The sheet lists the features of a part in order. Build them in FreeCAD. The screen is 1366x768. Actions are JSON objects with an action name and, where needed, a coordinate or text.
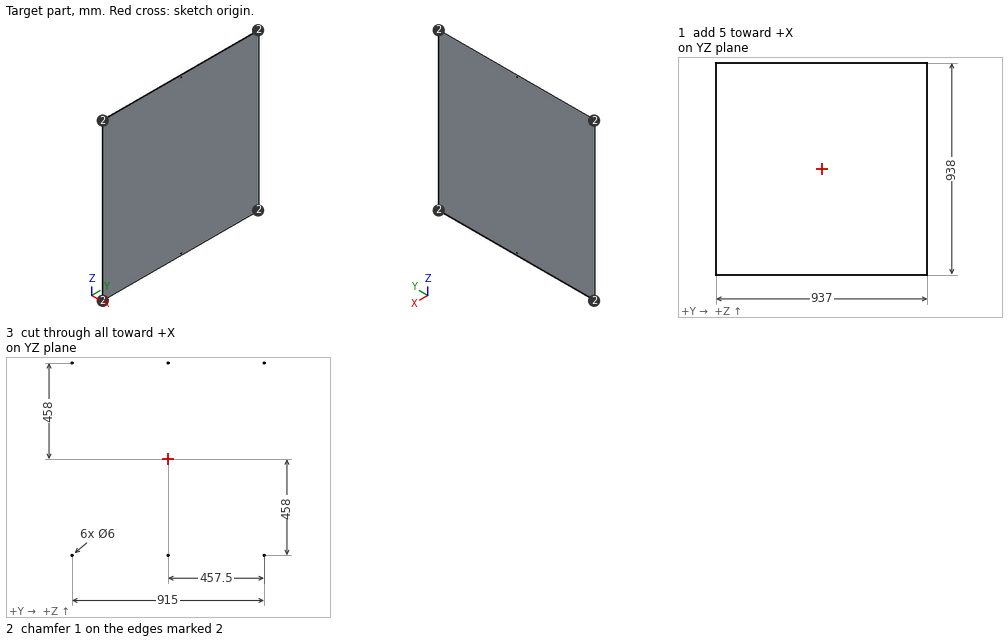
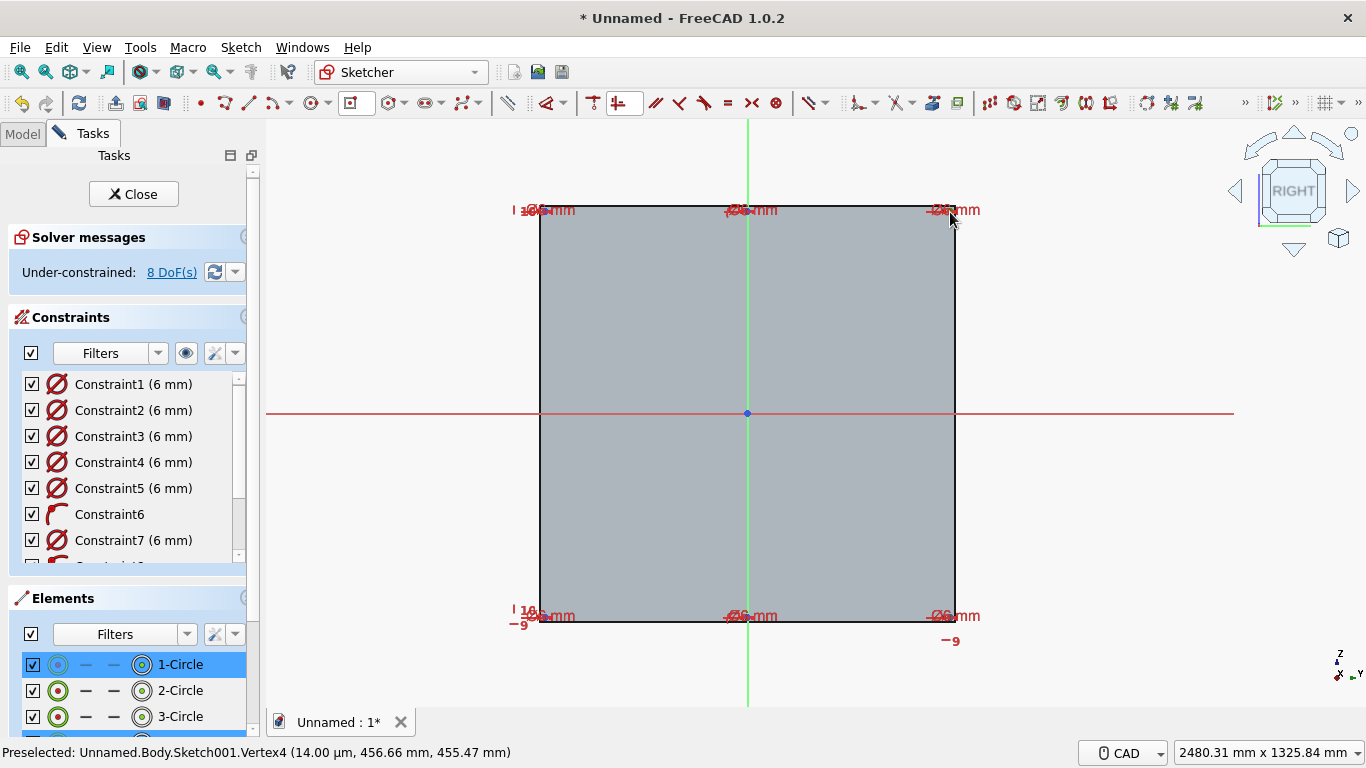
{"action": "key", "text": "v"}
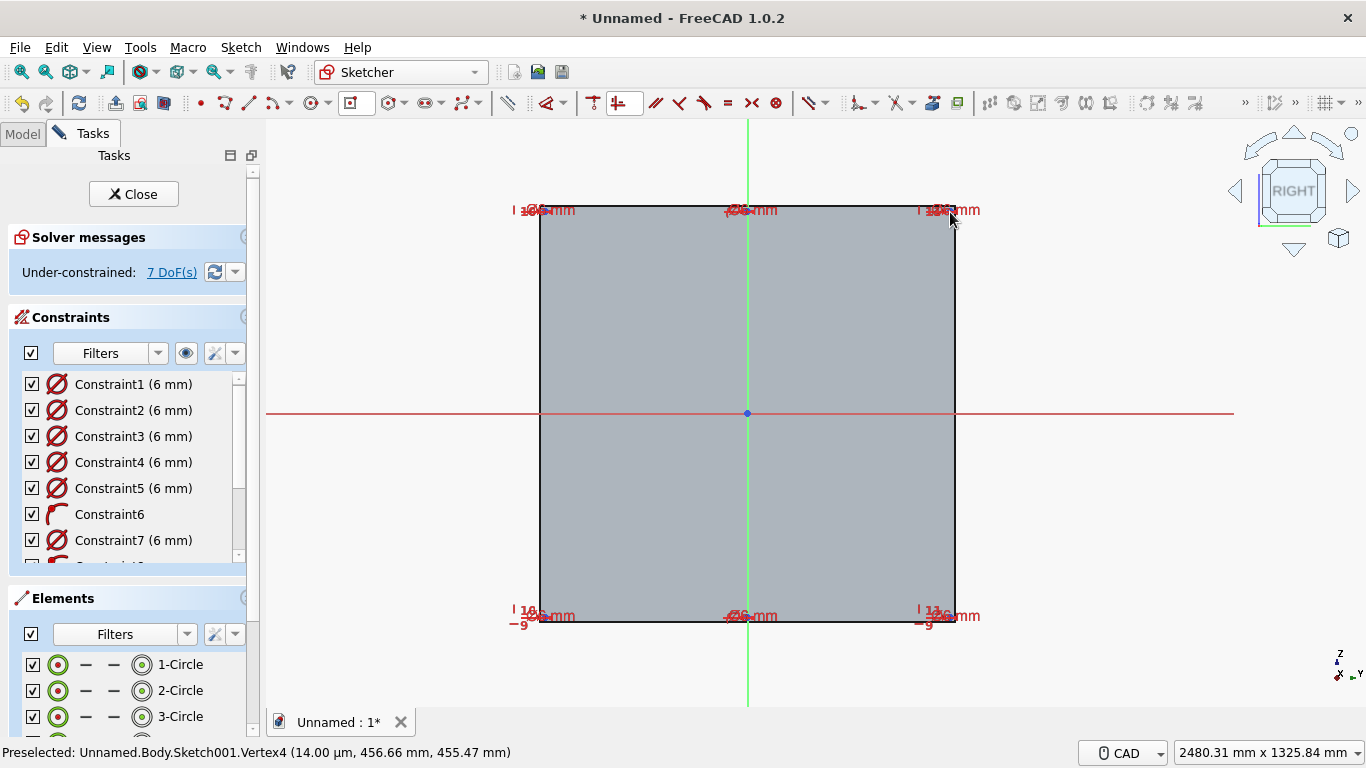
{"action": "left_click", "coordinate": [545, 212]}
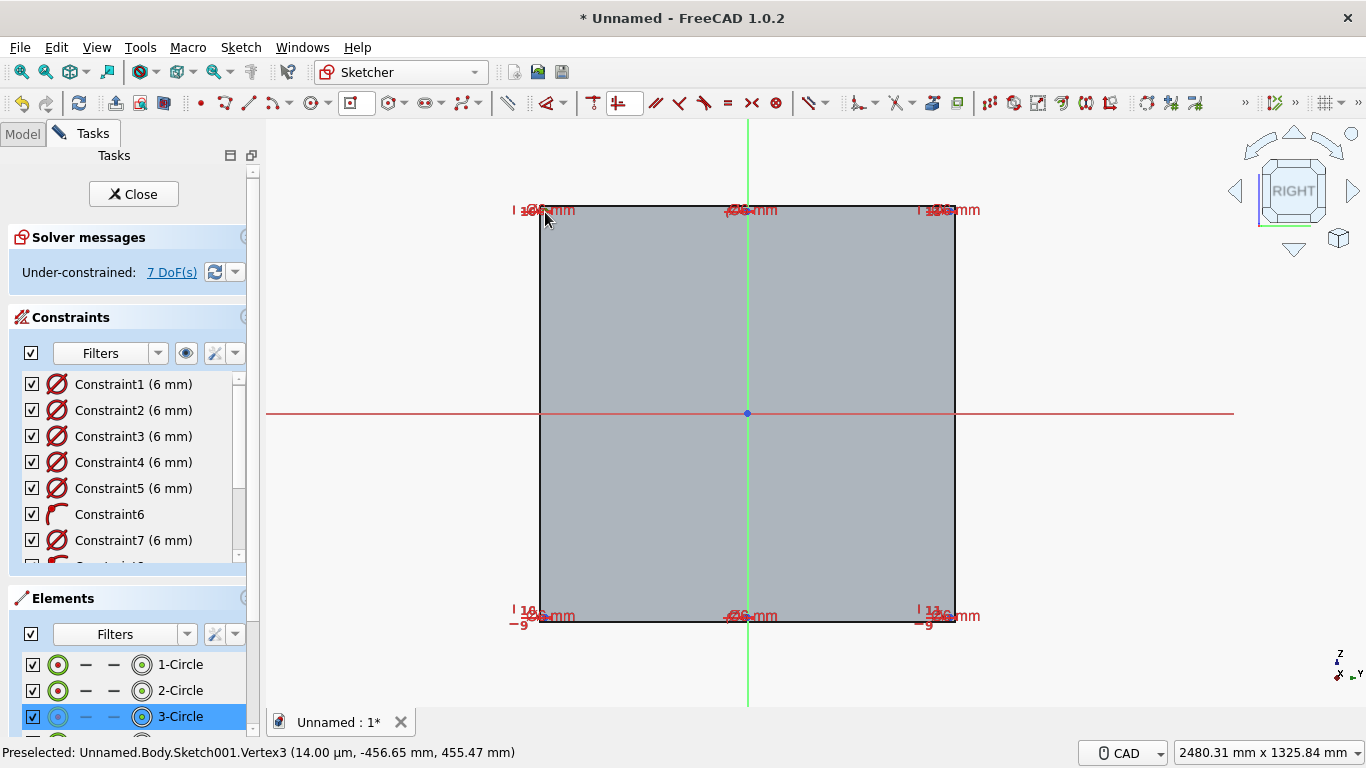
{"action": "left_click", "coordinate": [950, 212]}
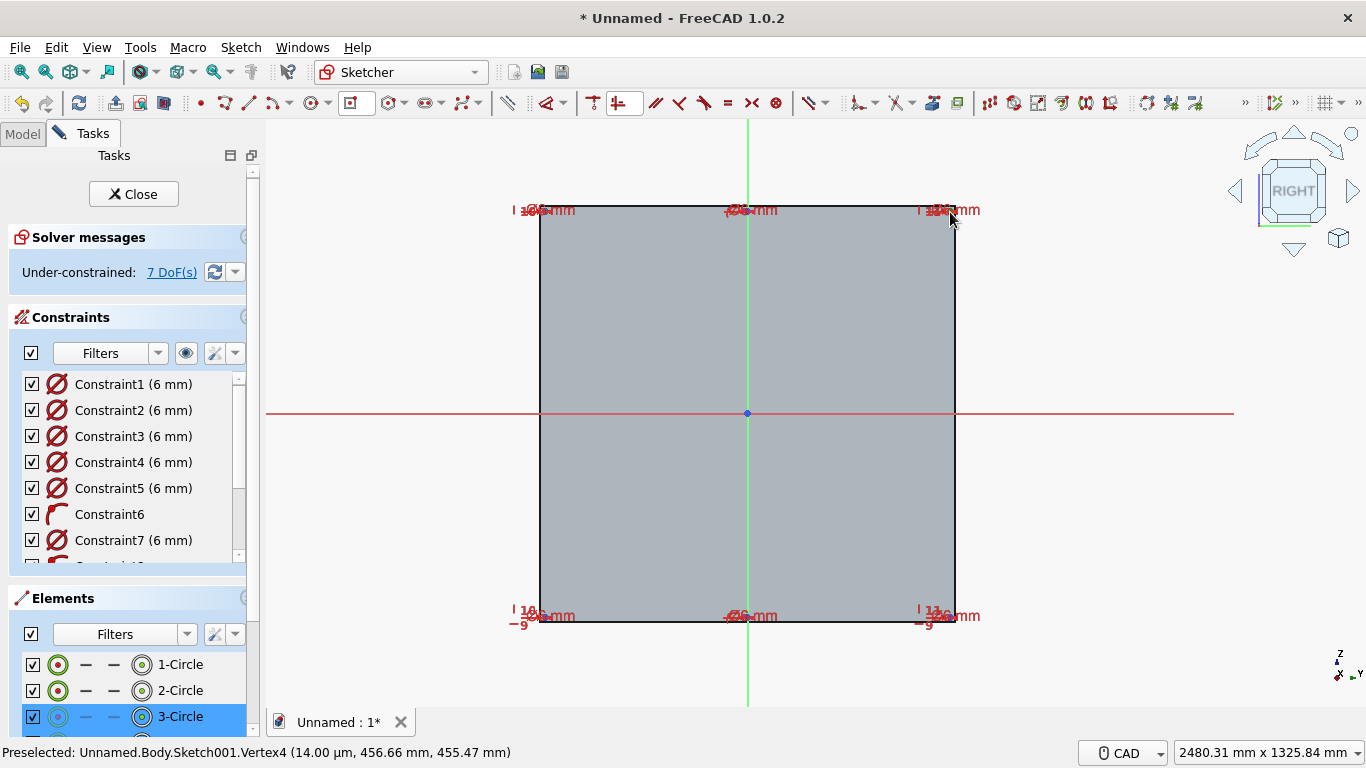
{"action": "key", "text": "h"}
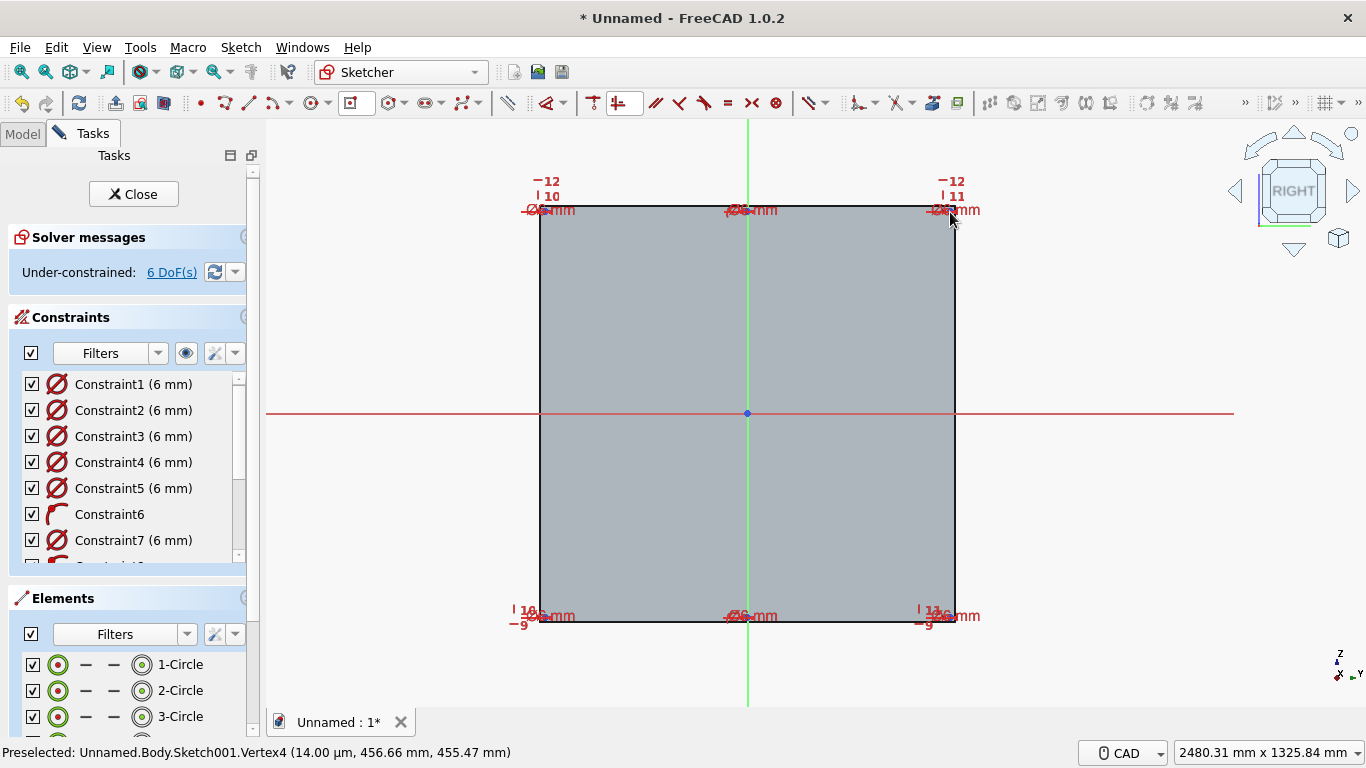
{"action": "left_click", "coordinate": [545, 212]}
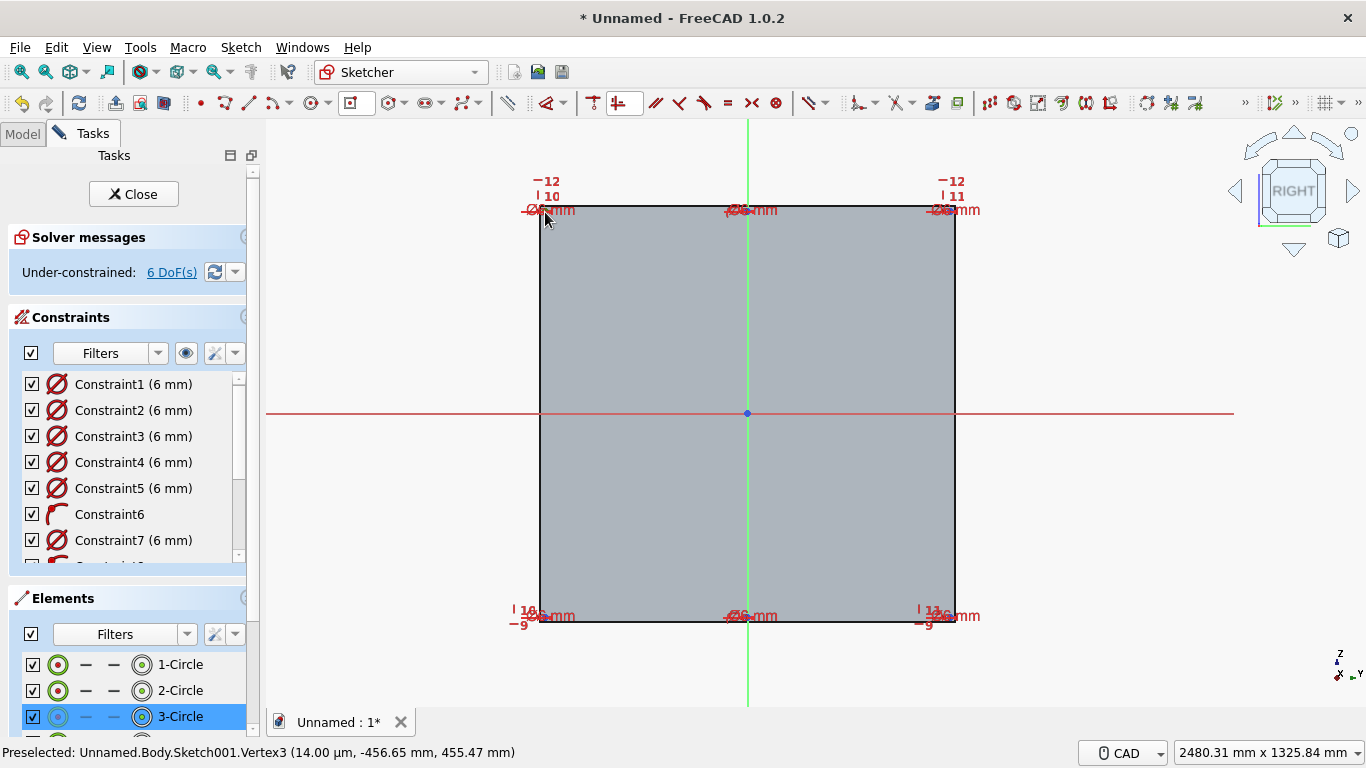
{"action": "left_click", "coordinate": [748, 212]}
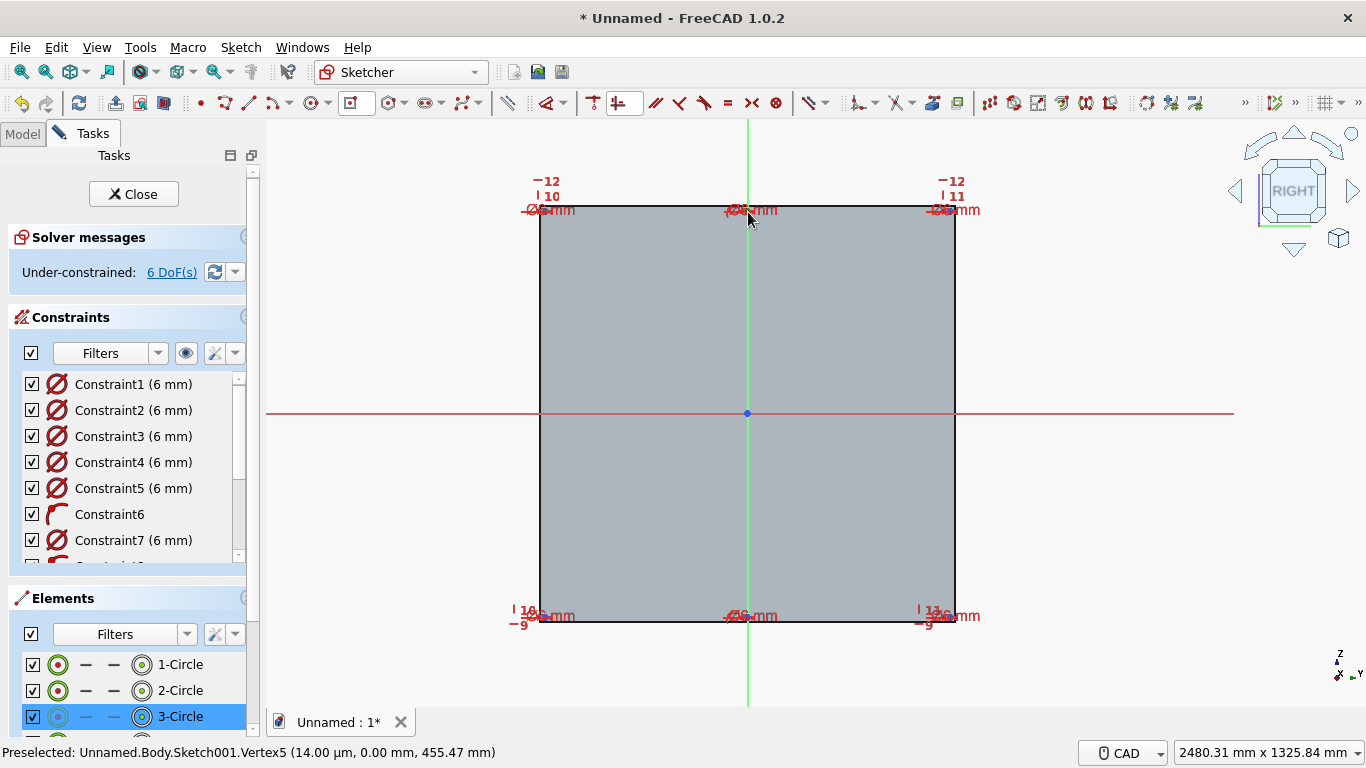
{"action": "key", "text": "h"}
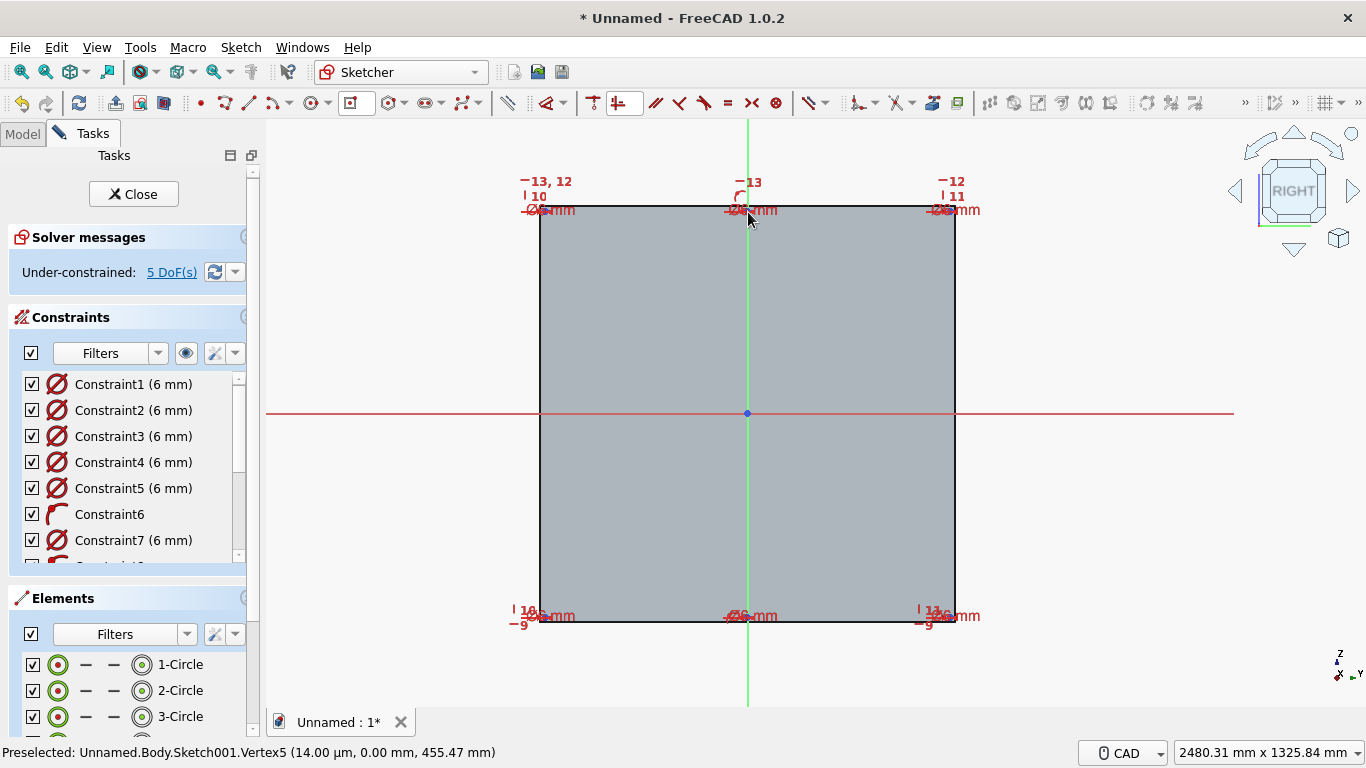
{"action": "left_click", "coordinate": [950, 618]}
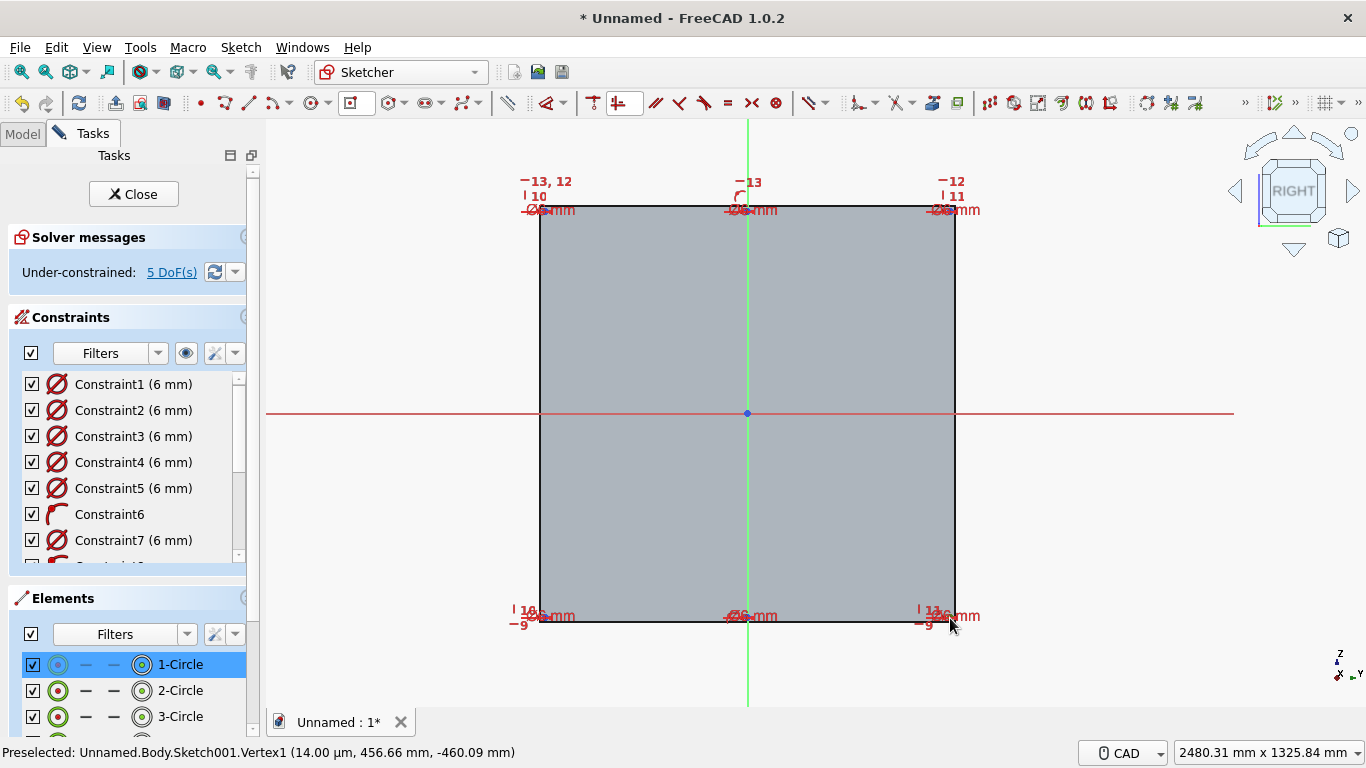
{"action": "left_click", "coordinate": [748, 618]}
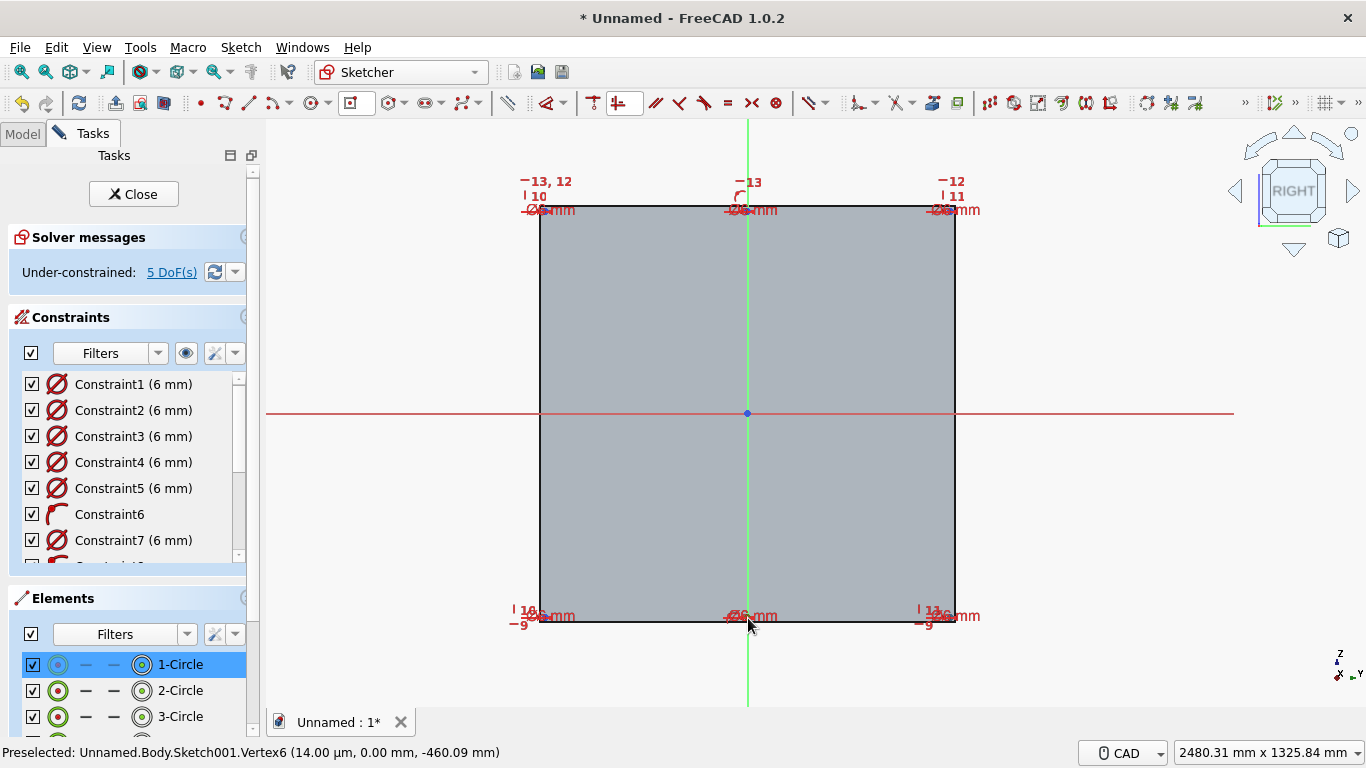
{"action": "left_click", "coordinate": [638, 104]}